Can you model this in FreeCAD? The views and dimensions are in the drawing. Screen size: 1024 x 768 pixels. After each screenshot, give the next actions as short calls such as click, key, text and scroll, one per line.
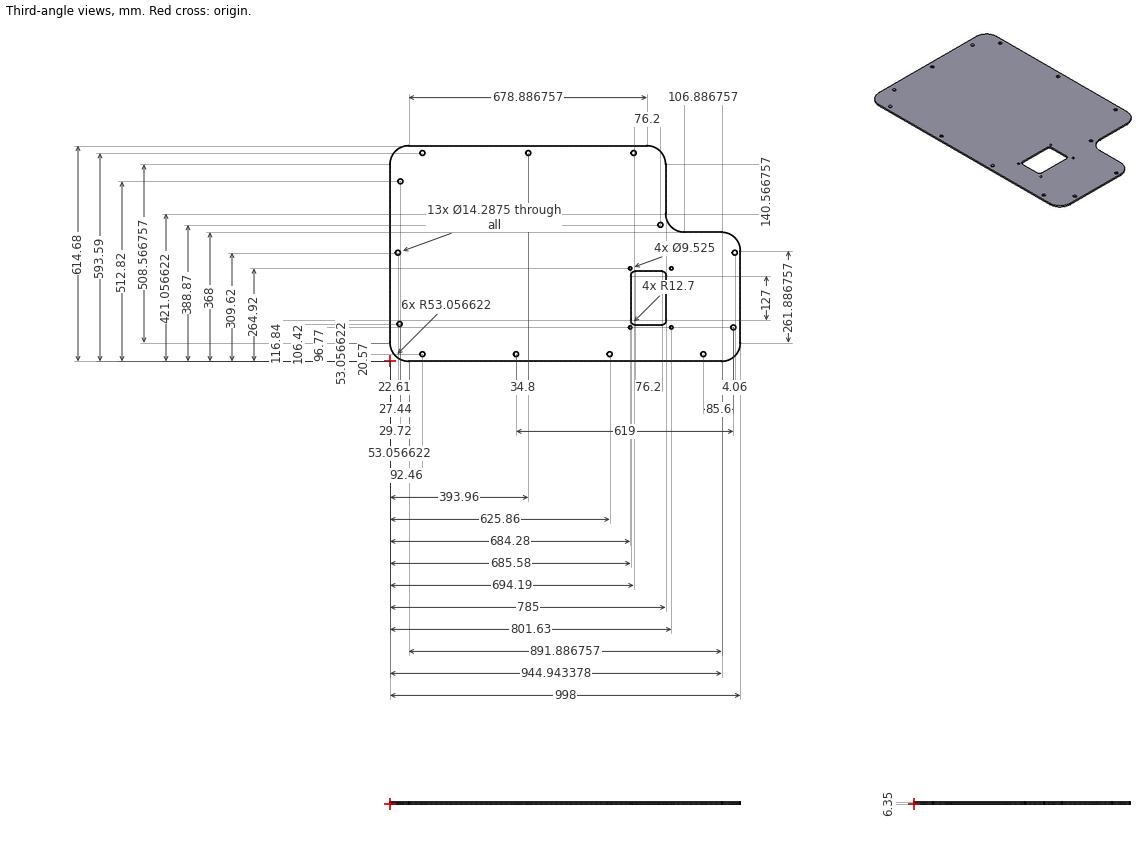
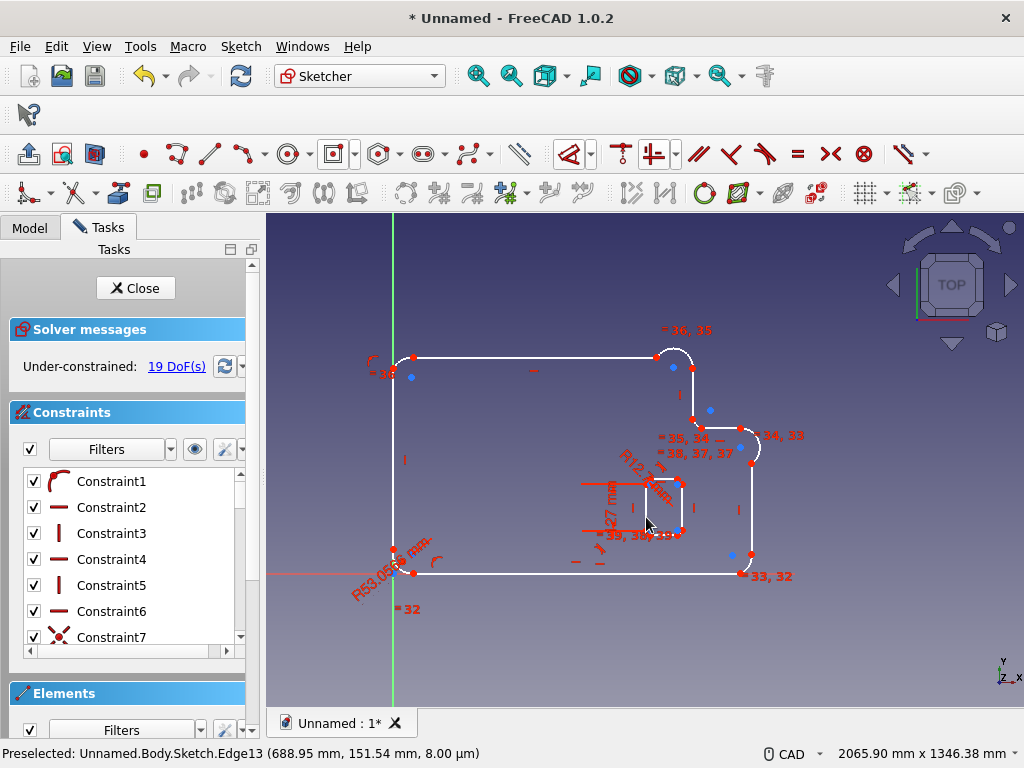
scroll(662, 479, up, 2)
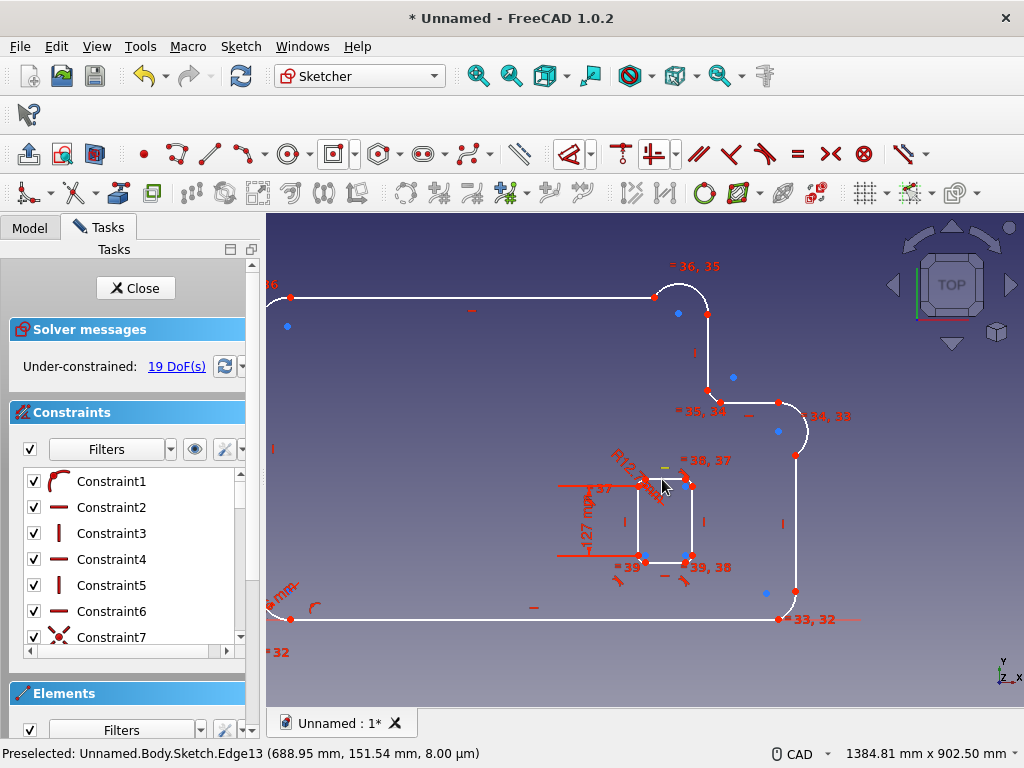
click(661, 479)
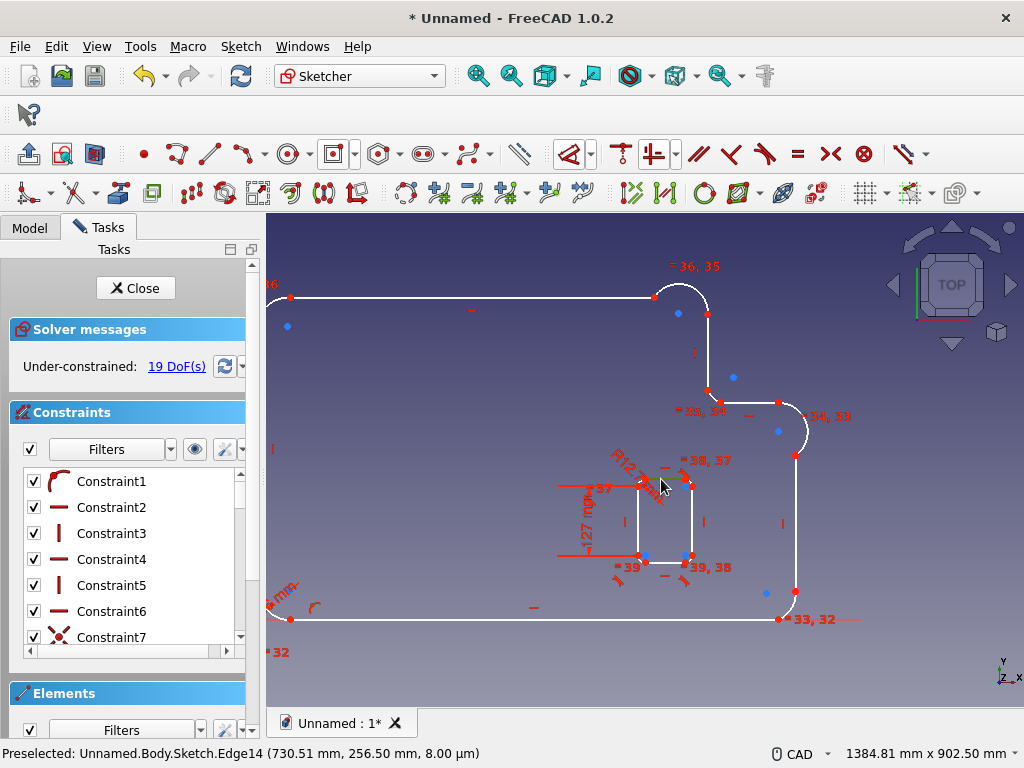
click(590, 154)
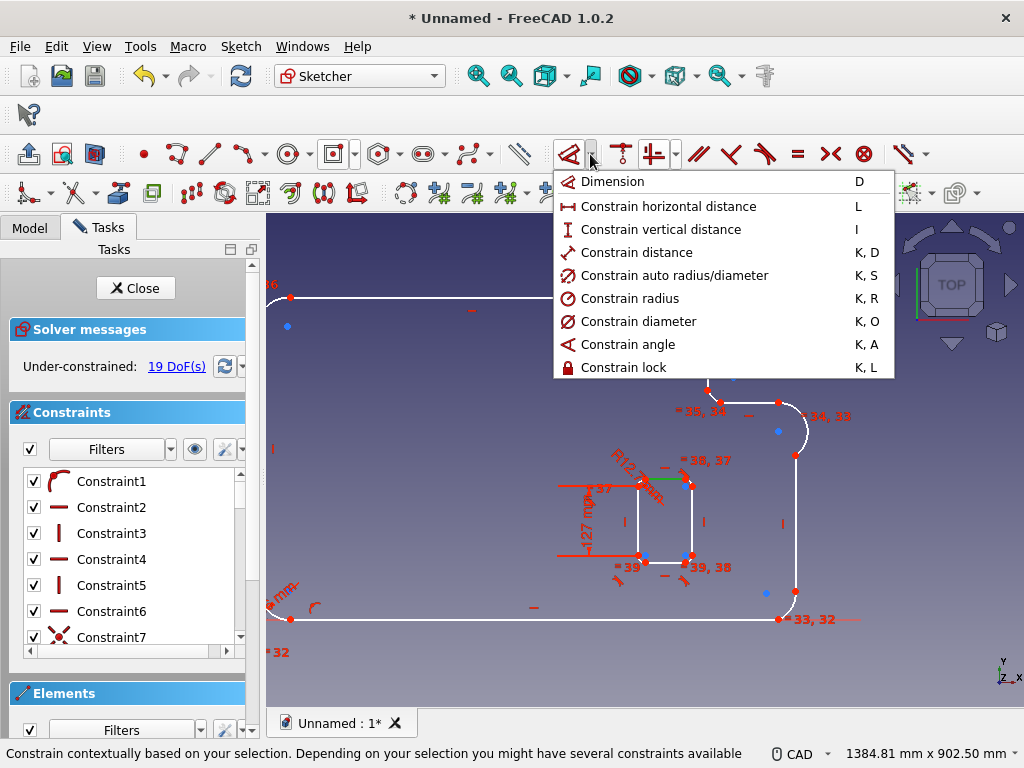
click(724, 206)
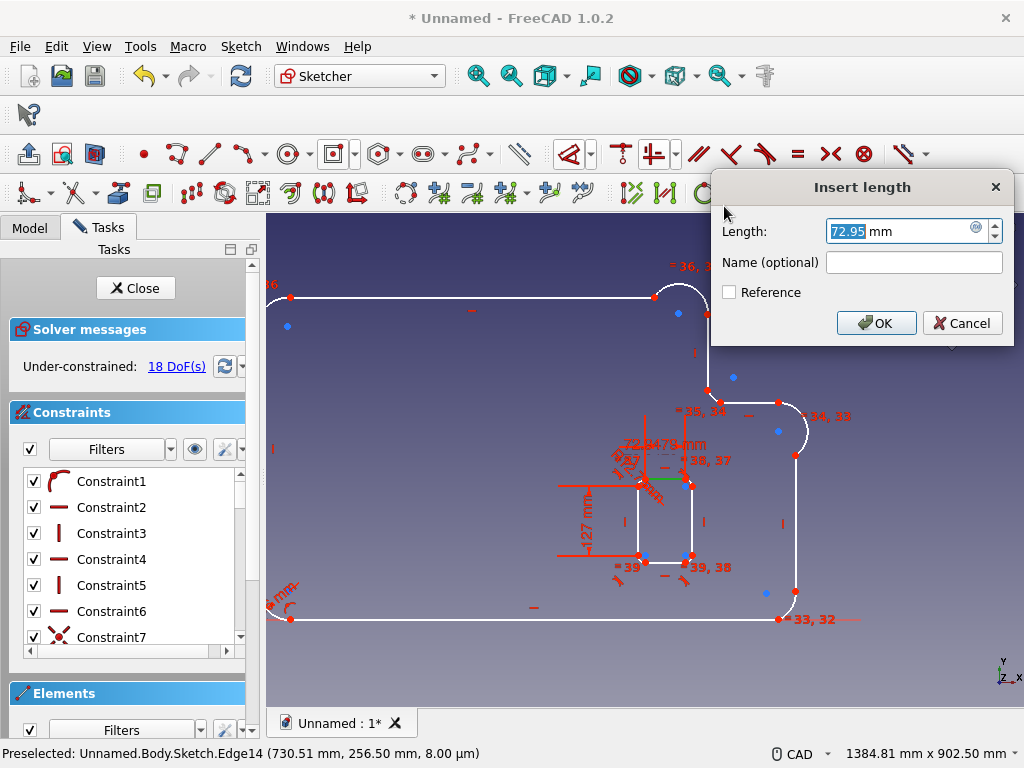
text(76.2)
key(Return)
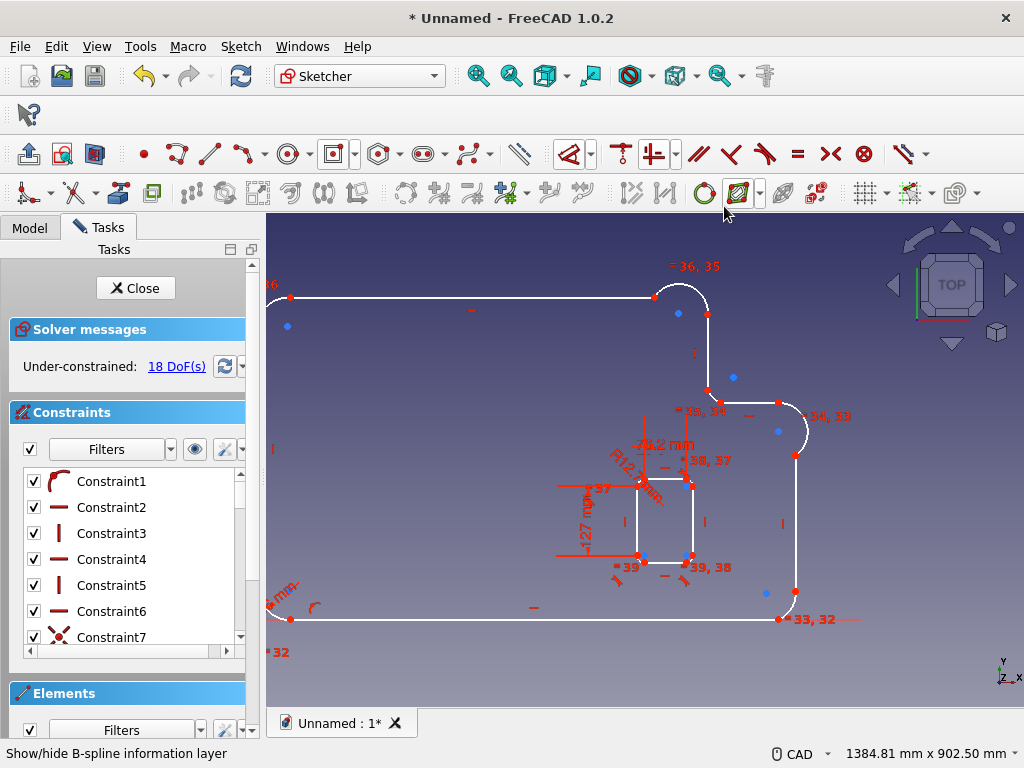
click(796, 592)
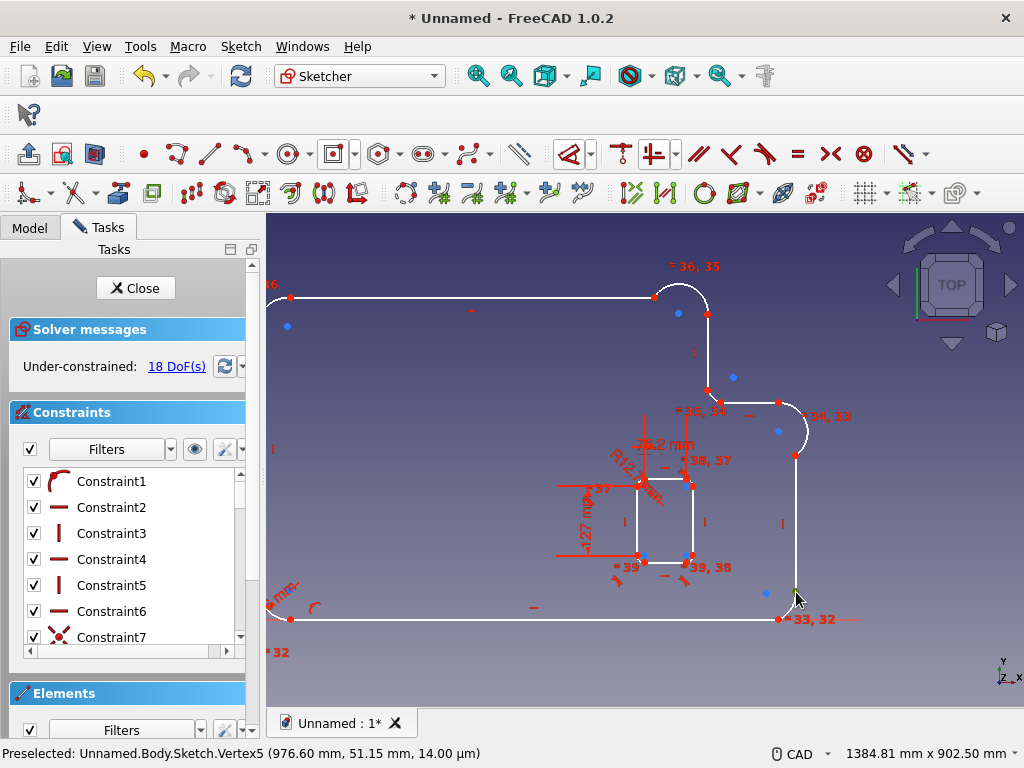
click(590, 154)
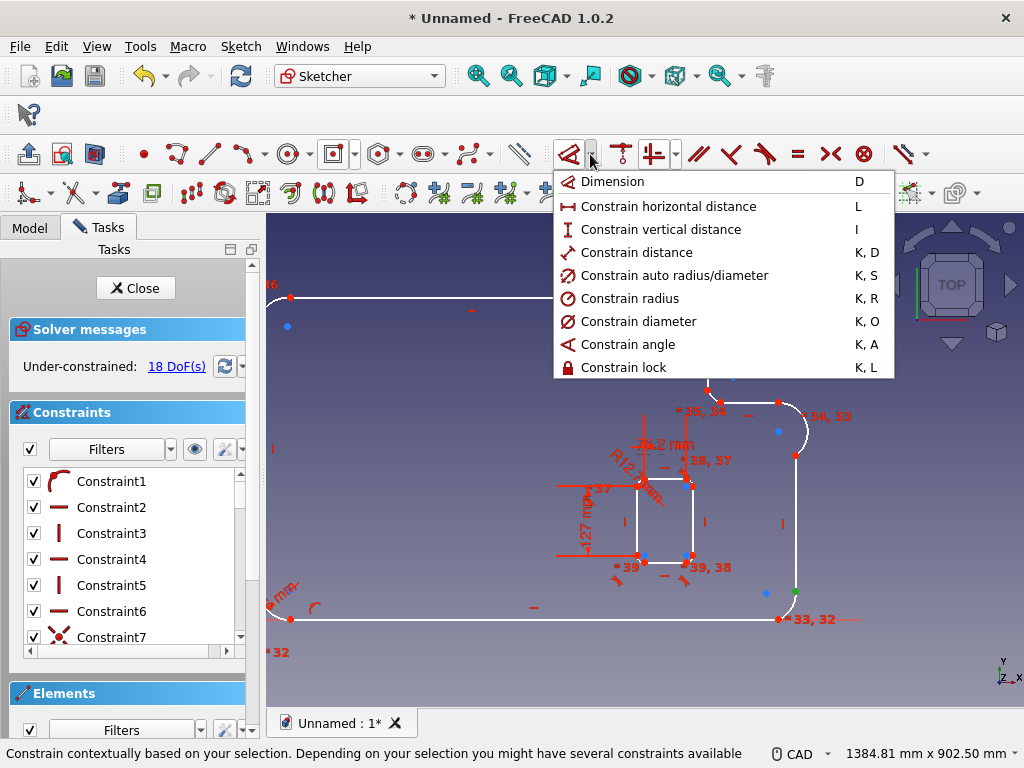
click(724, 206)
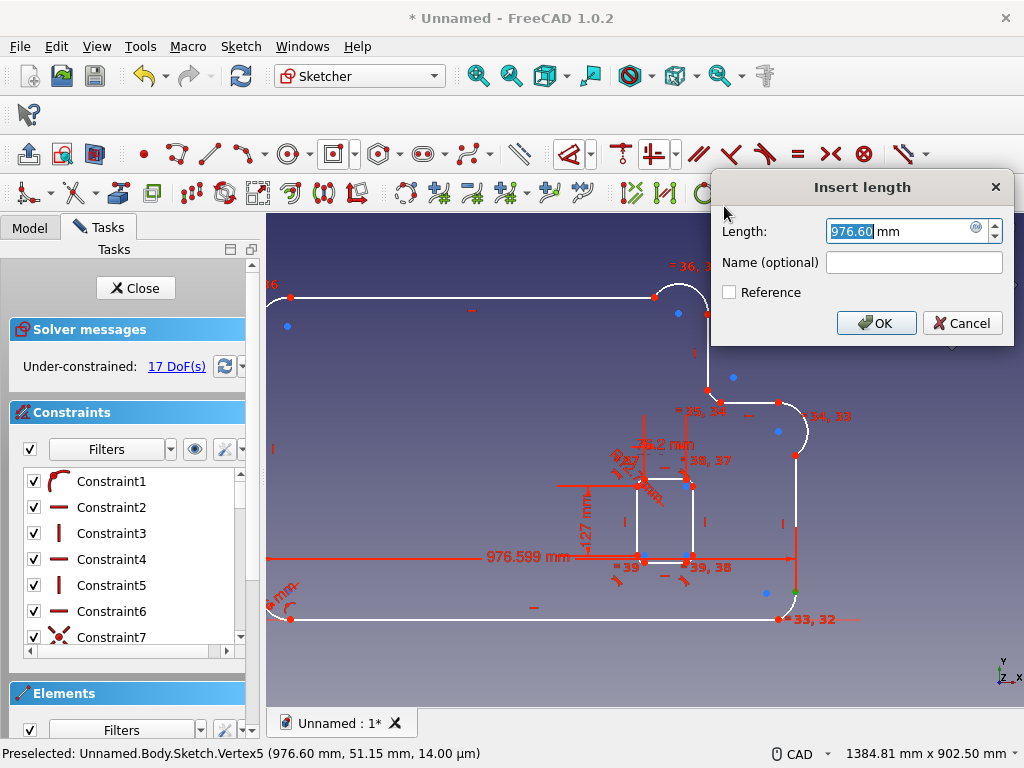
text(998)
key(Return)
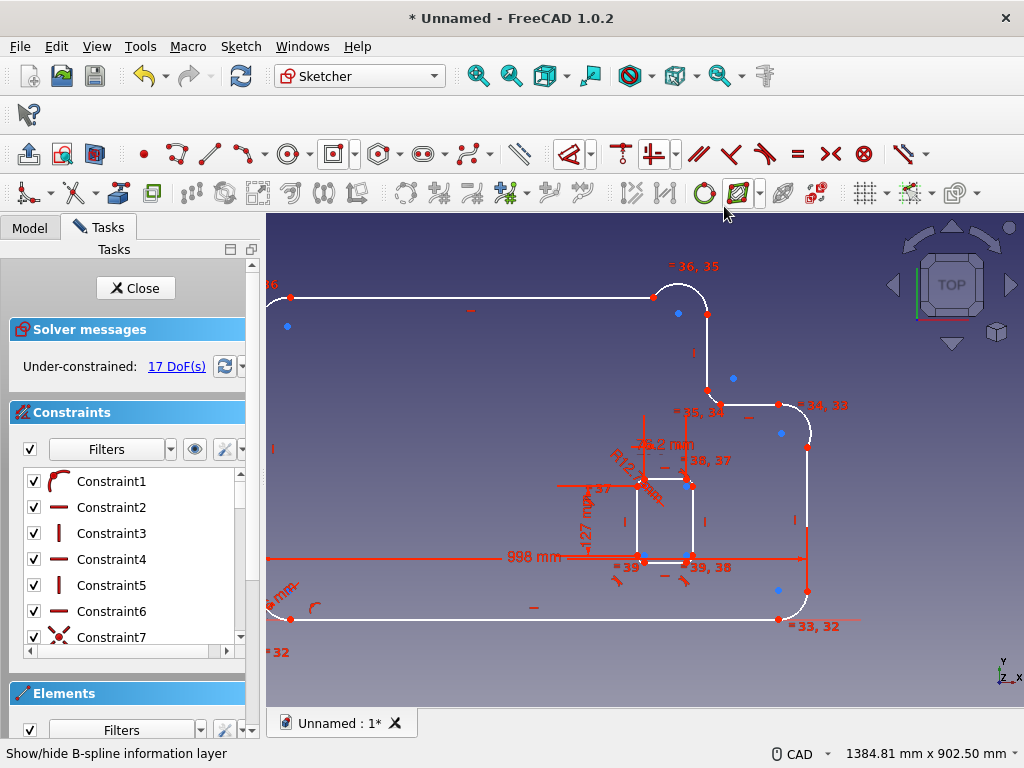
click(778, 405)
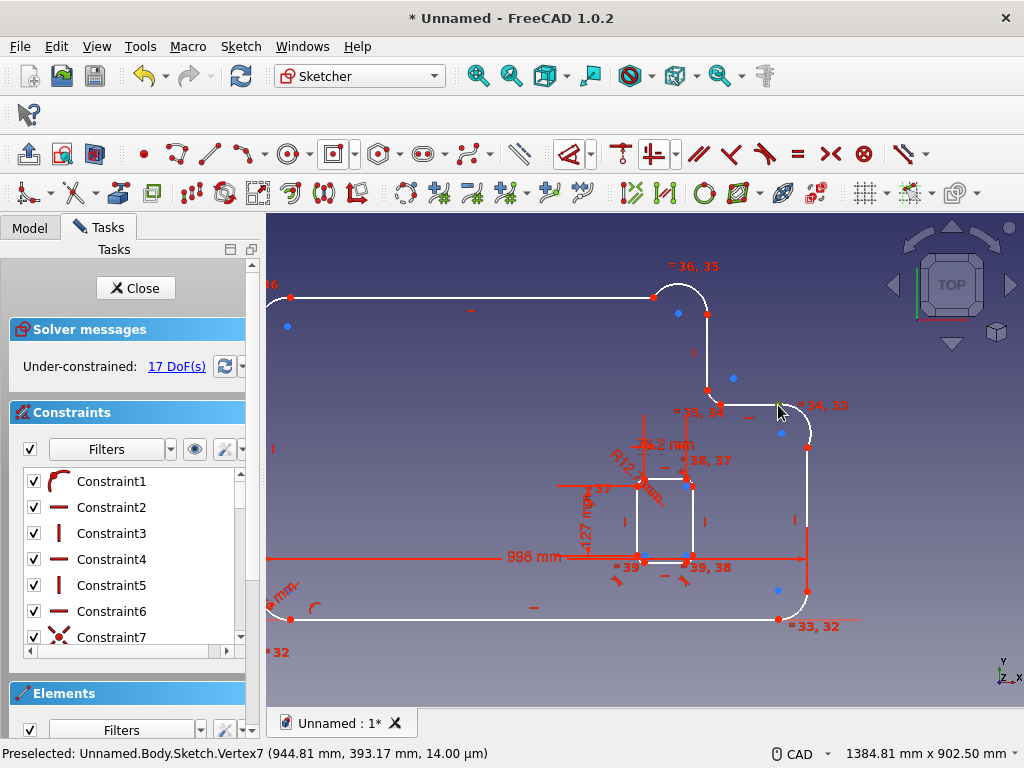
key(i)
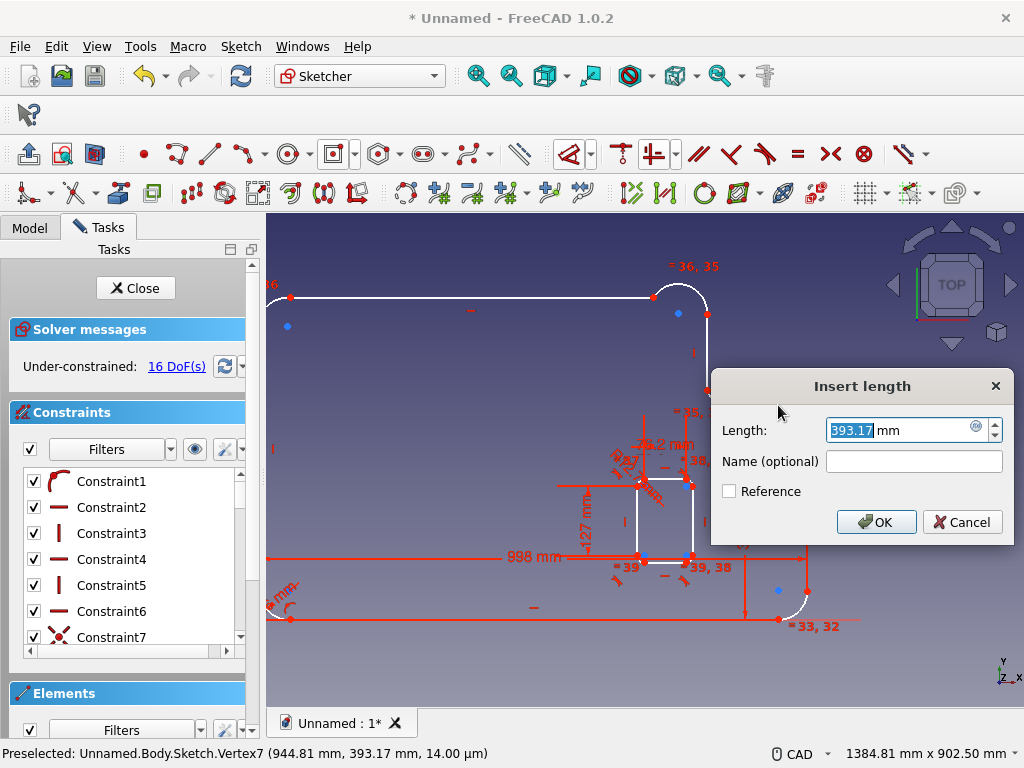
text(368)
key(Return)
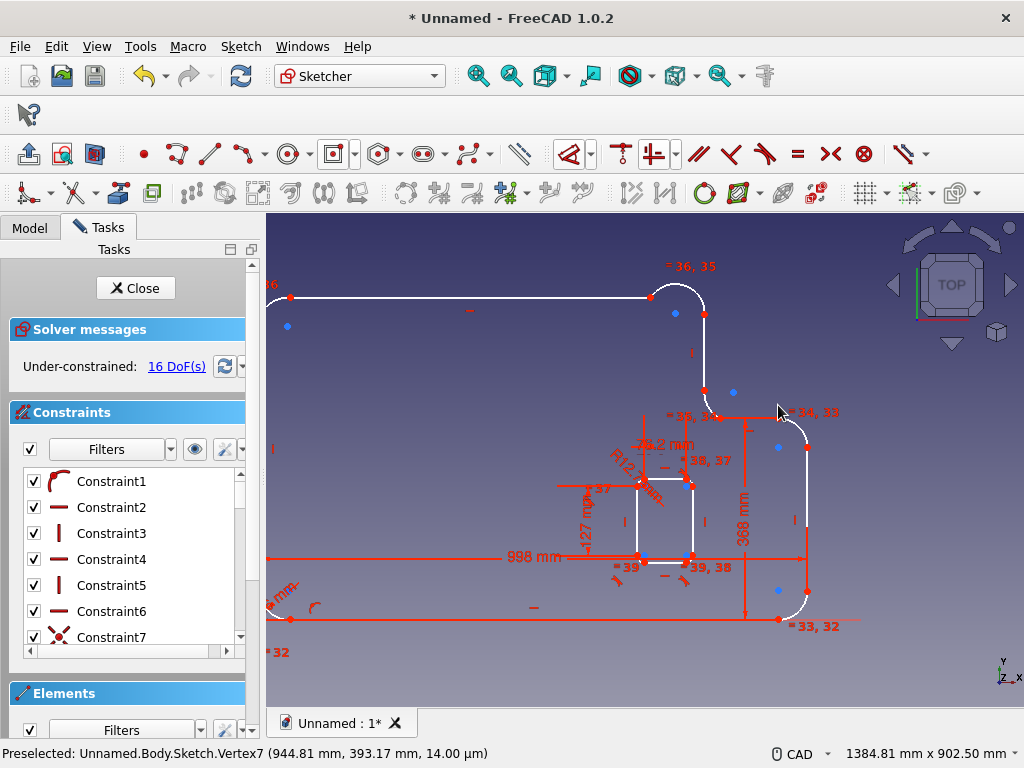
click(704, 391)